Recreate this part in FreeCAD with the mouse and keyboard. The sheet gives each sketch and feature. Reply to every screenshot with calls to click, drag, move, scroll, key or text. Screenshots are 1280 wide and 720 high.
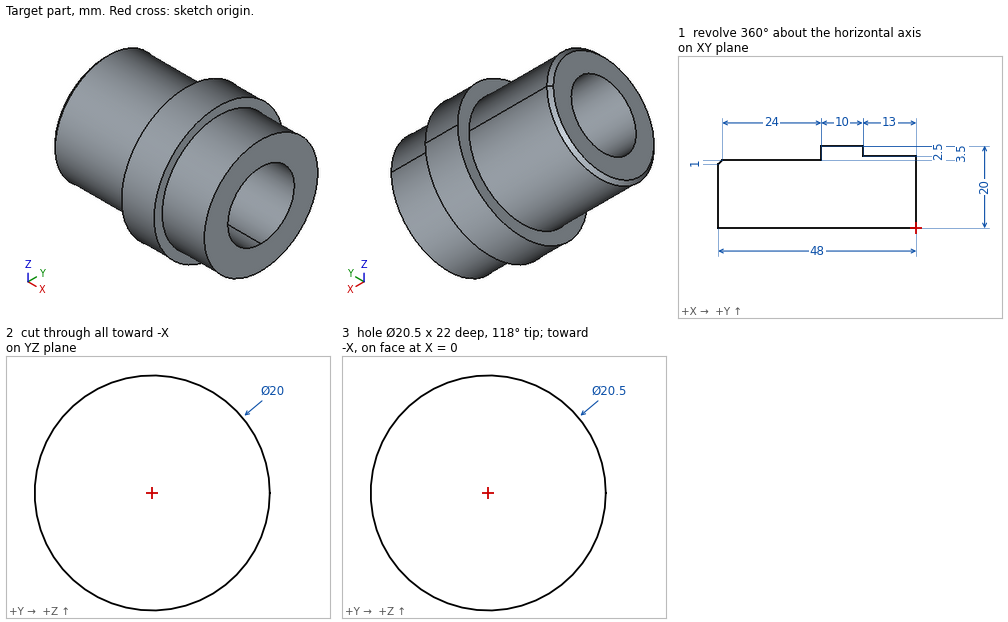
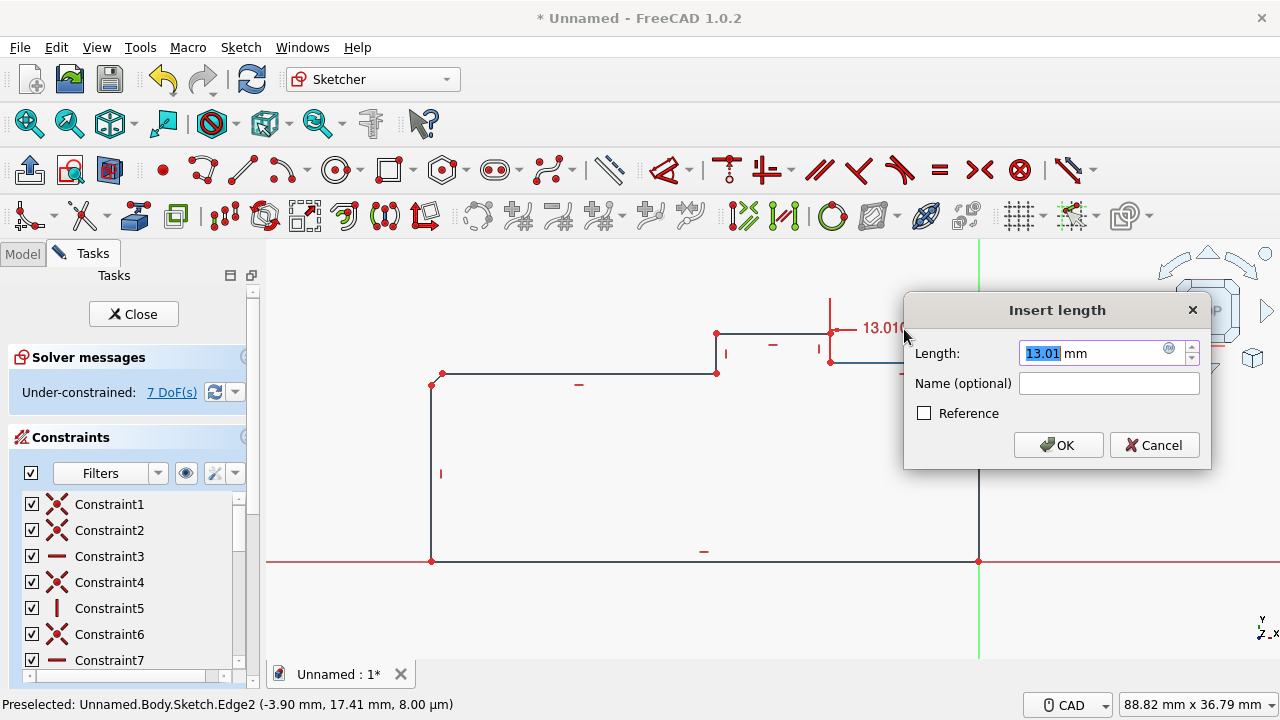
text(13)
key(Return)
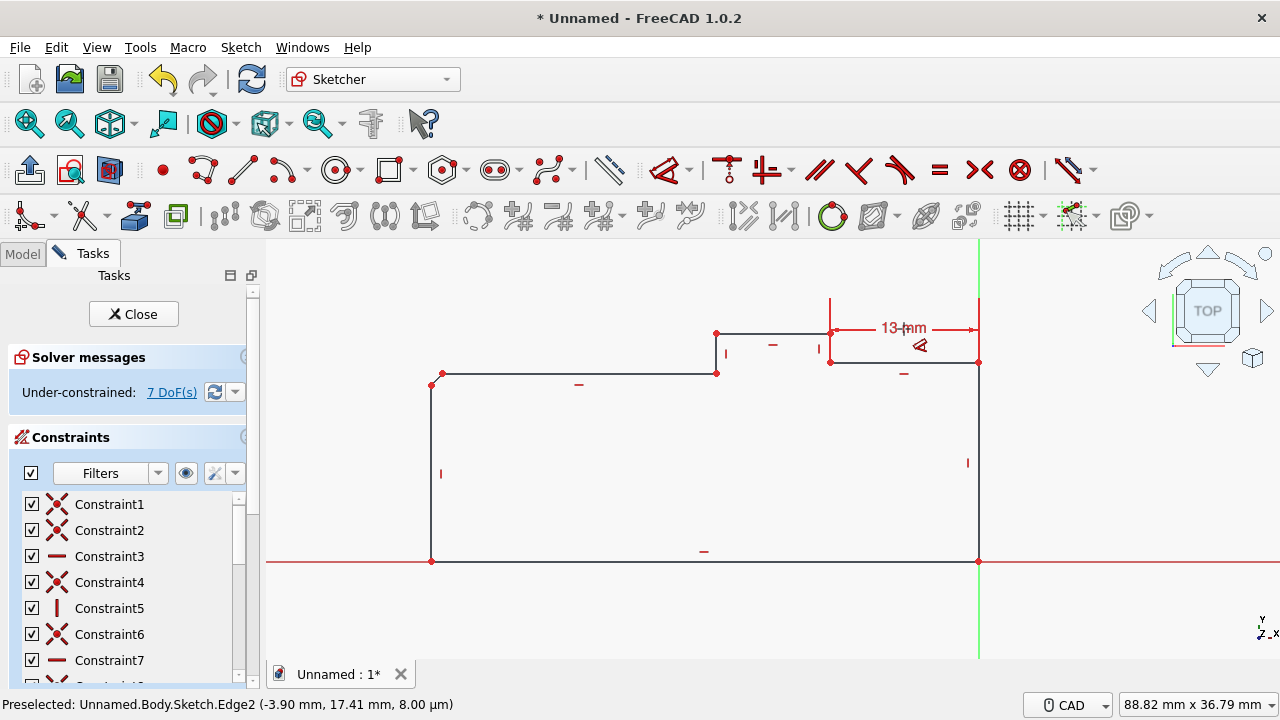
click(796, 334)
click(773, 300)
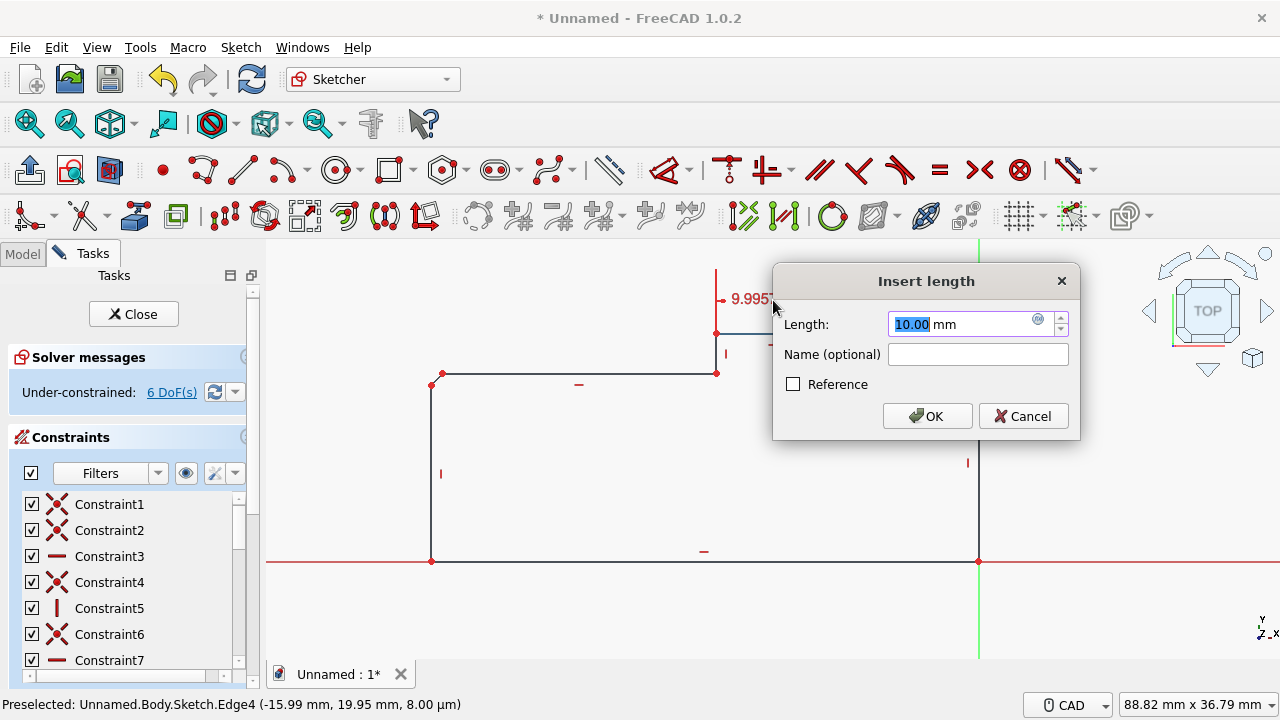
text(10)
key(Return)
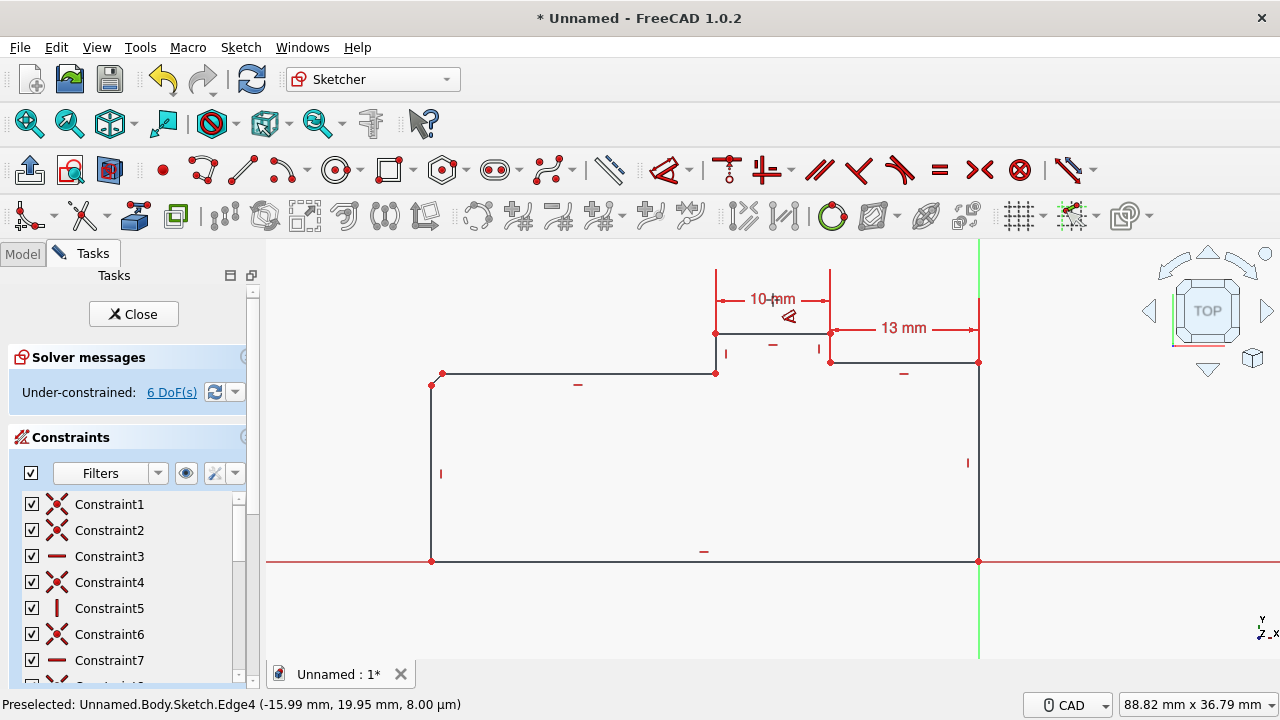
click(634, 374)
click(579, 340)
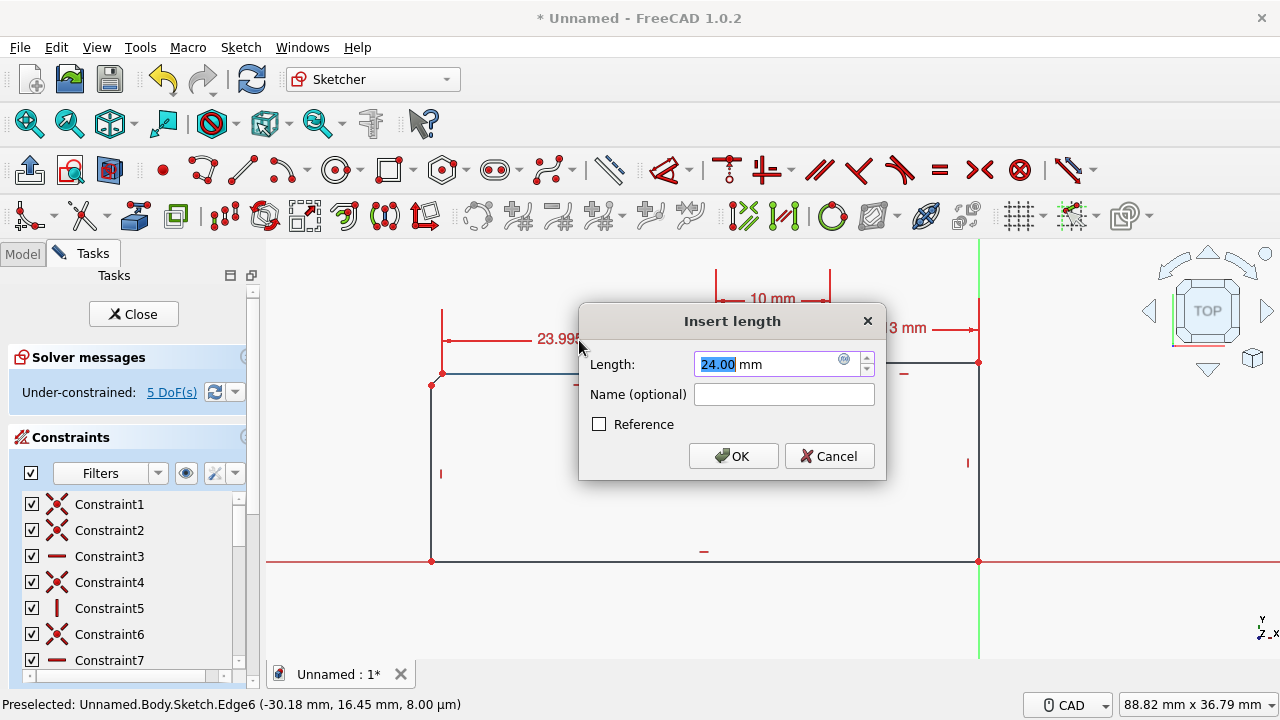
text(24)
key(Return)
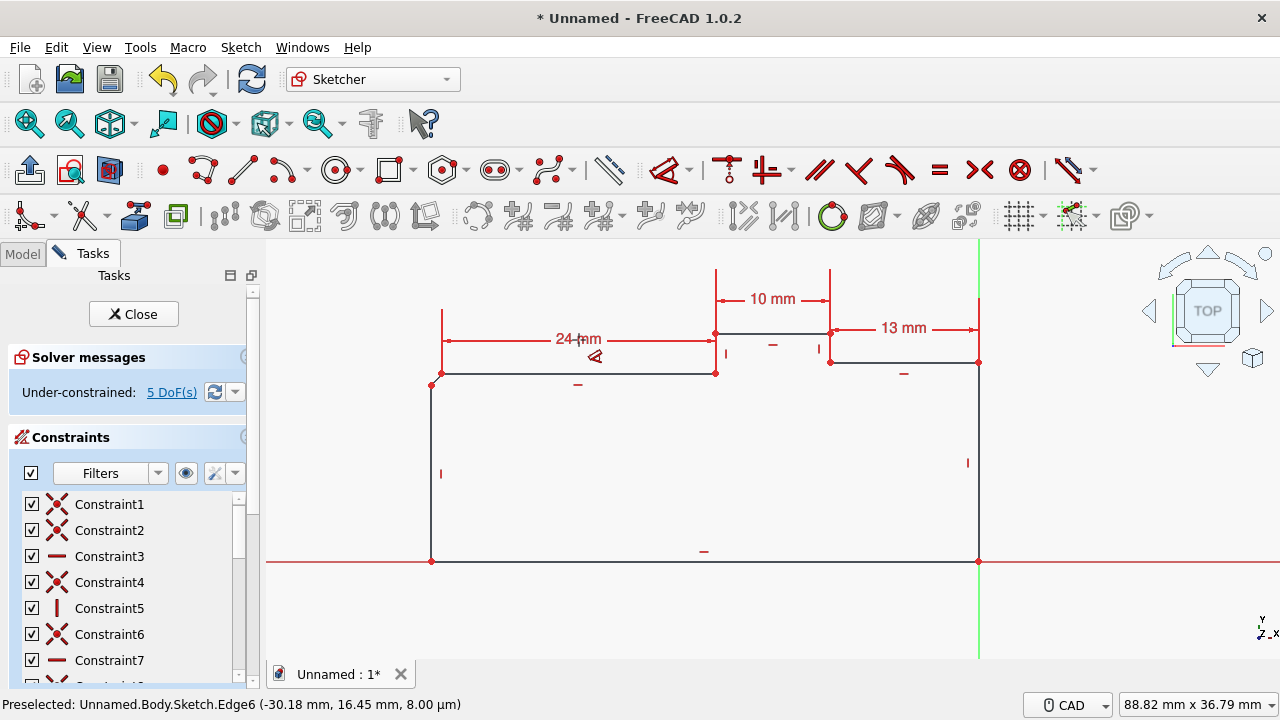
click(595, 562)
click(705, 596)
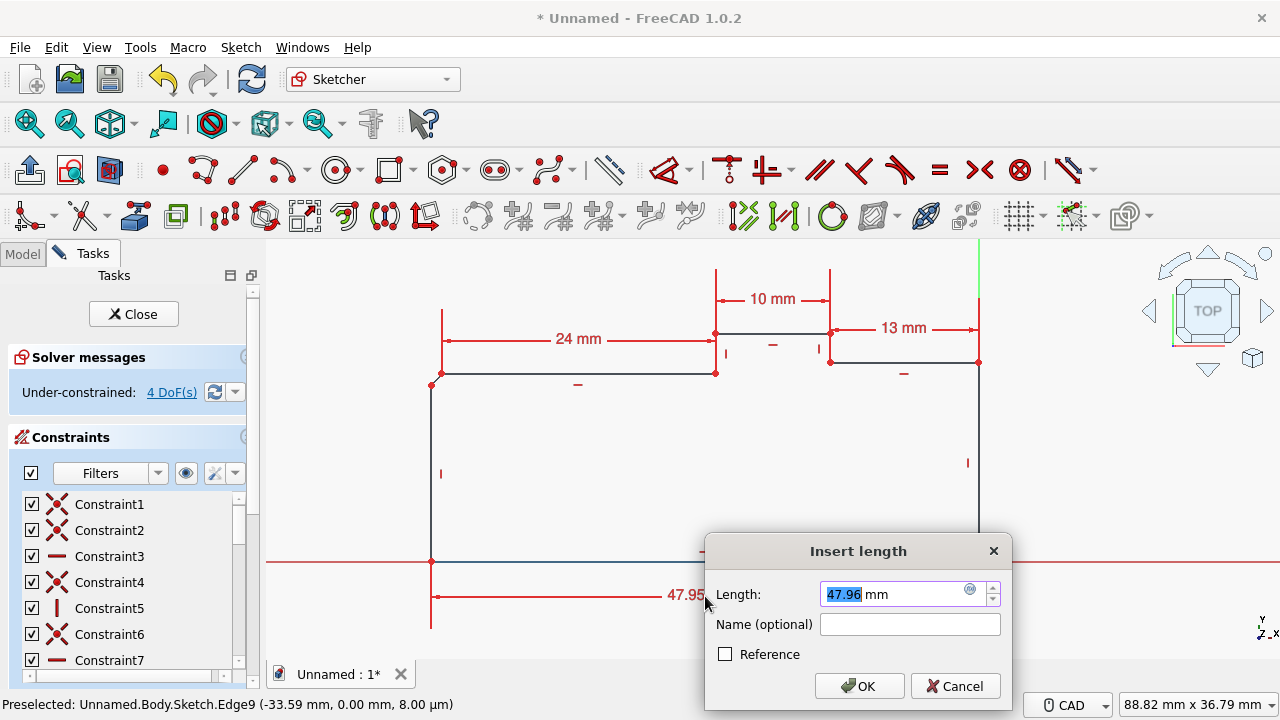
text(48)
key(Return)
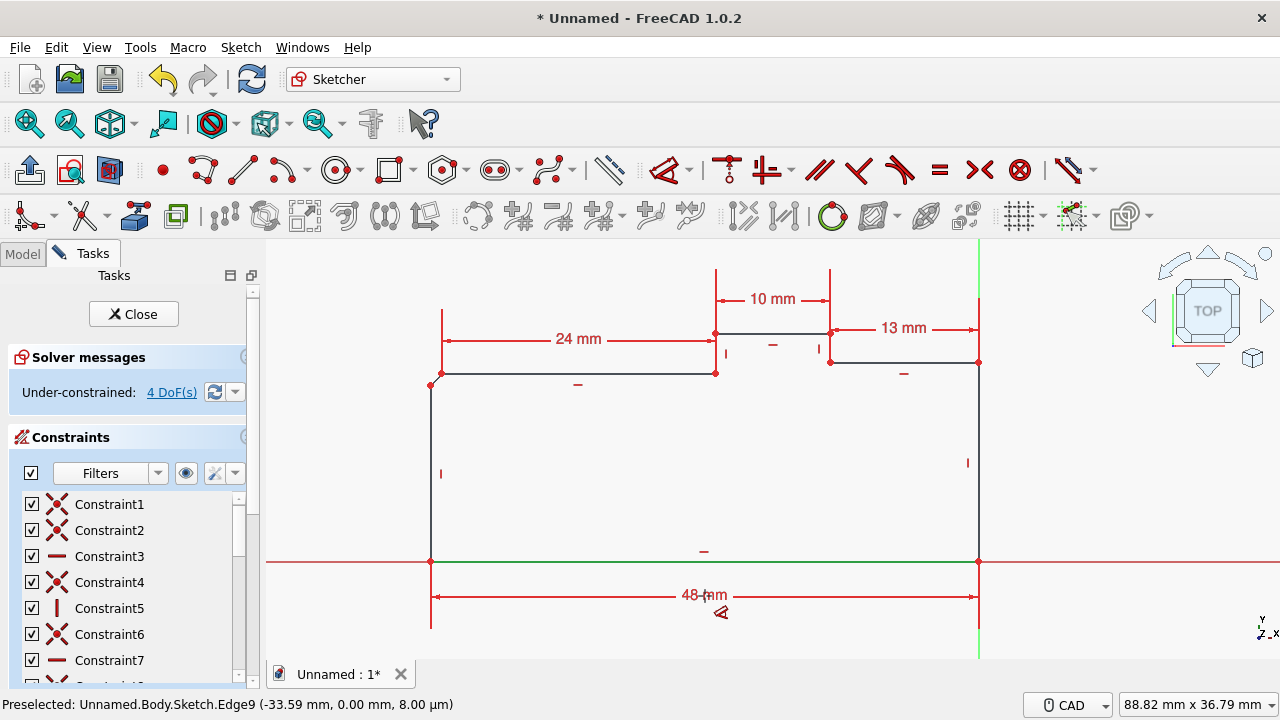
scroll(436, 380, up, 7)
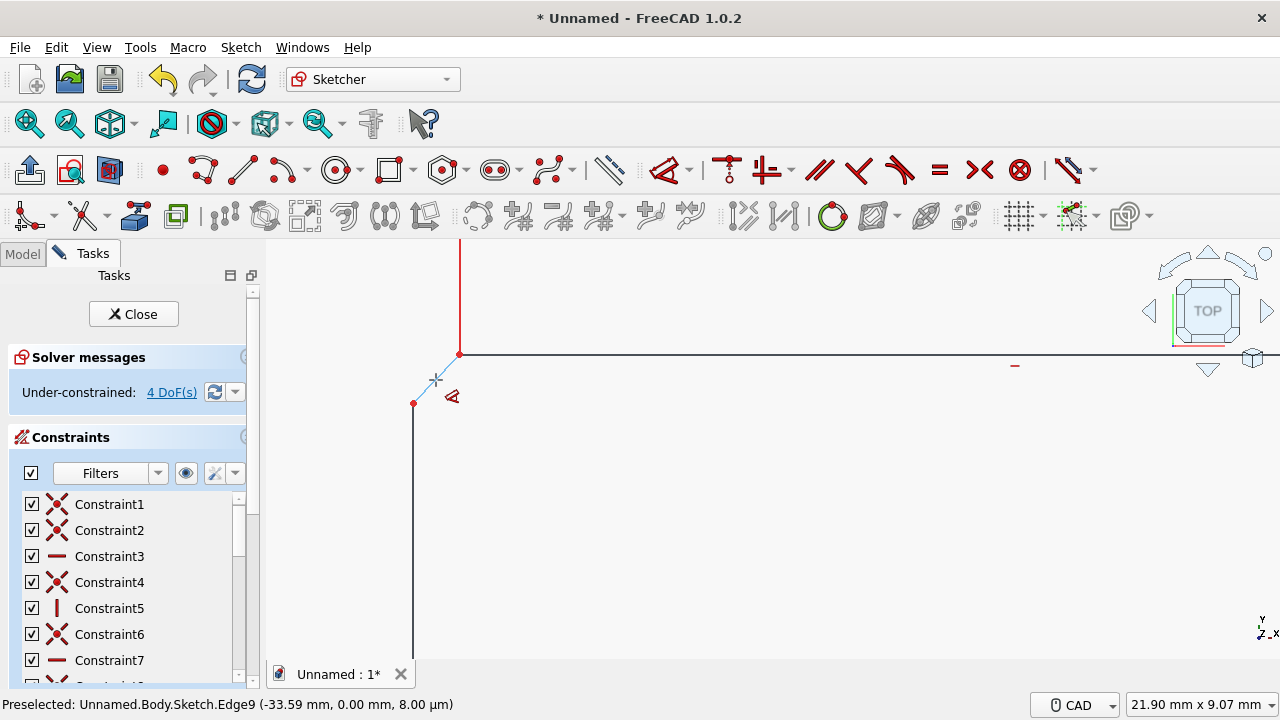
click(436, 379)
click(379, 379)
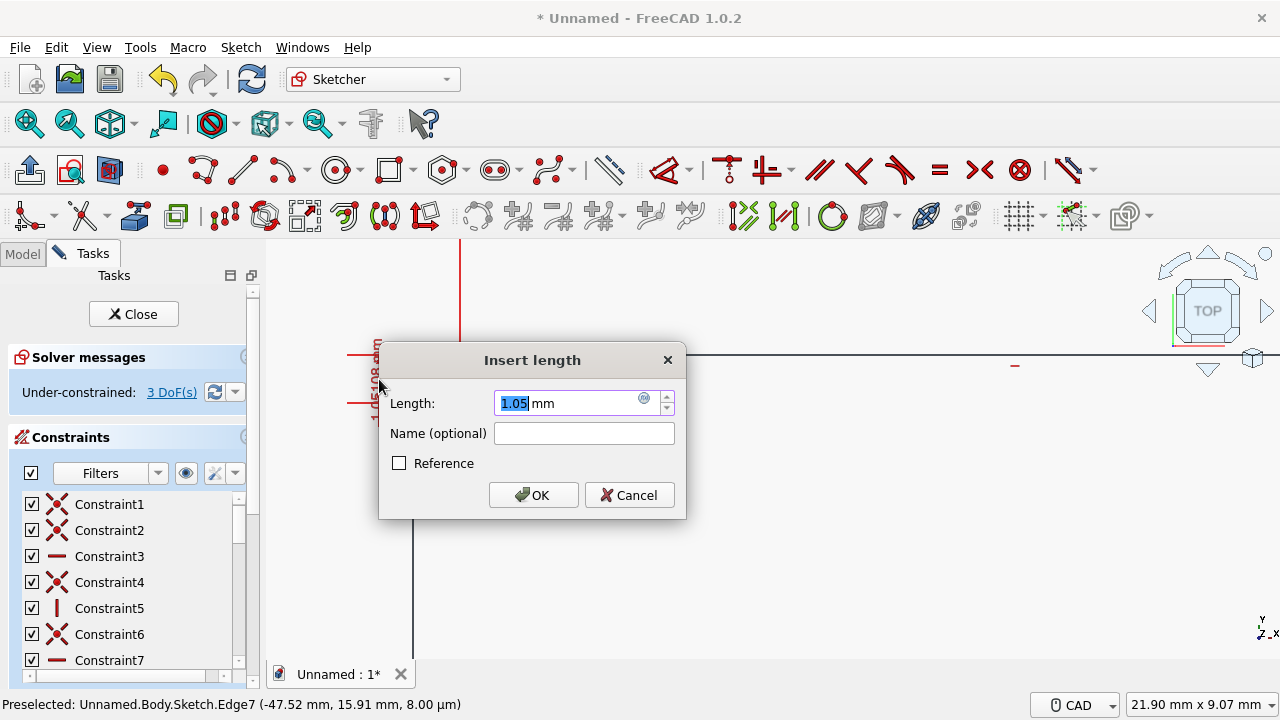
text(1)
key(Return)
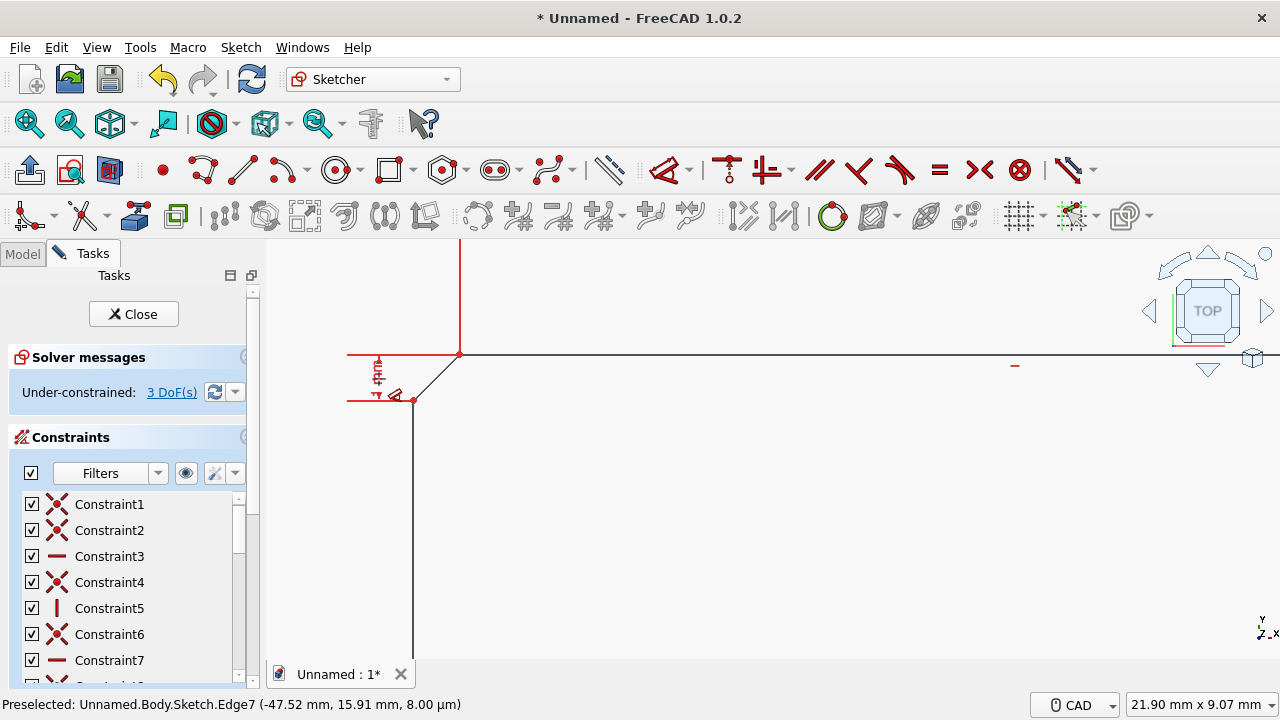
scroll(436, 382, down, 7)